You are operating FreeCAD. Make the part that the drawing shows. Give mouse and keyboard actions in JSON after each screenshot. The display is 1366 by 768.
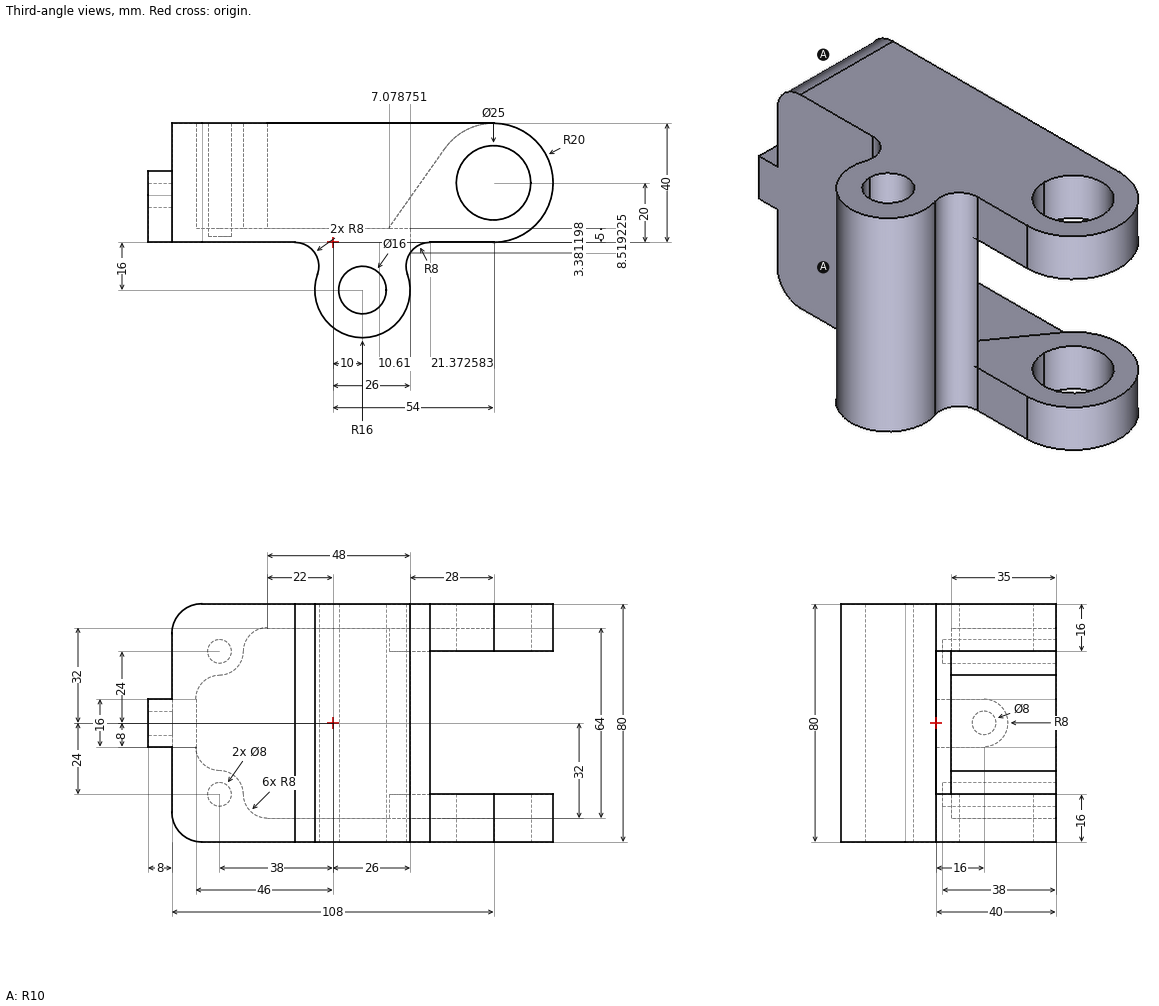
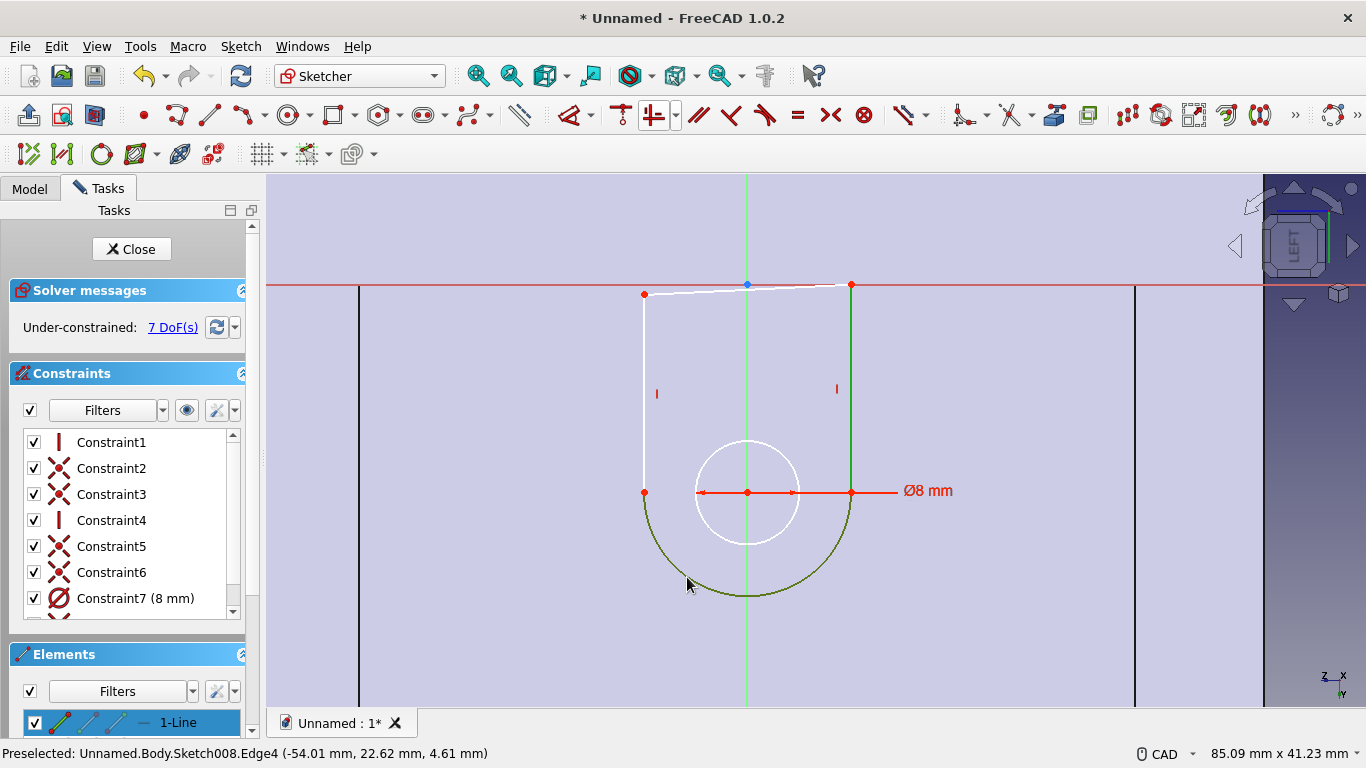
{"action": "key", "text": "t"}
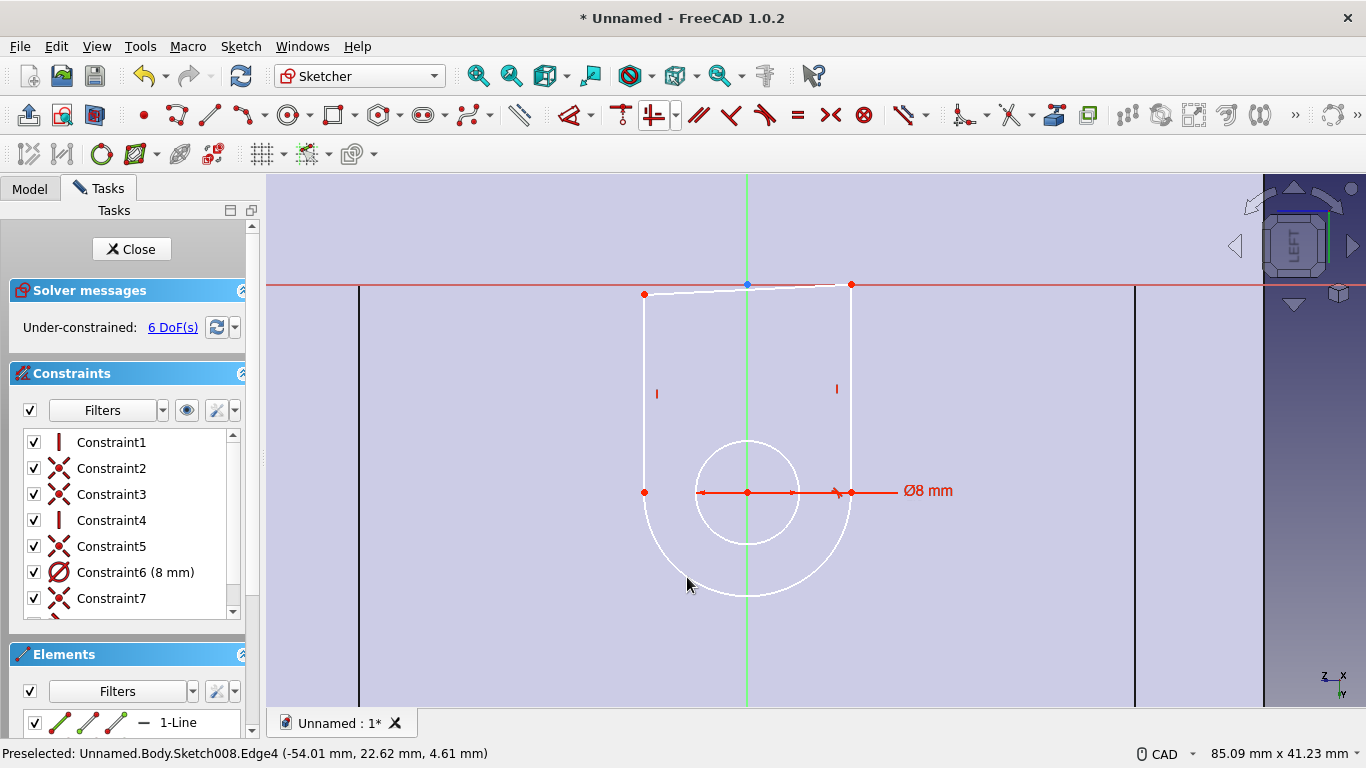
{"action": "left_click", "coordinate": [644, 354]}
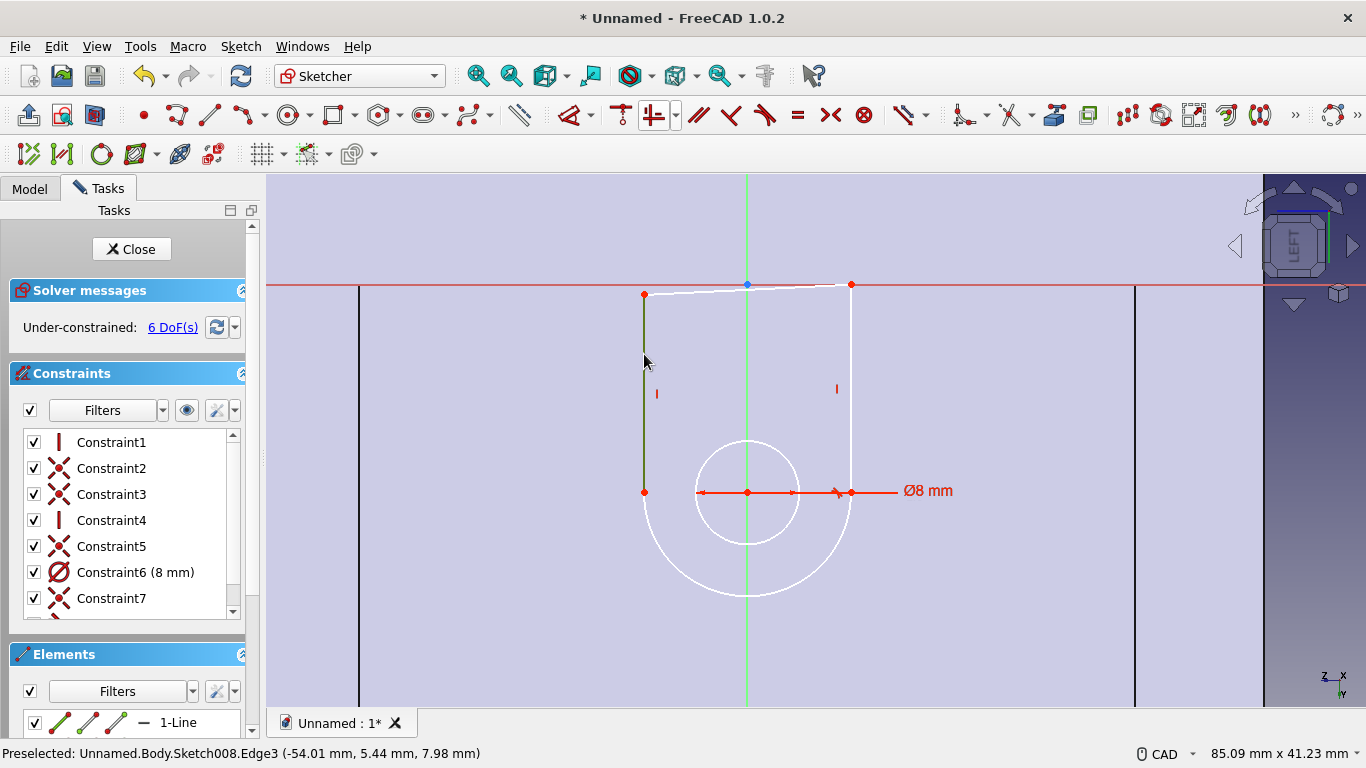
{"action": "left_click", "coordinate": [687, 577]}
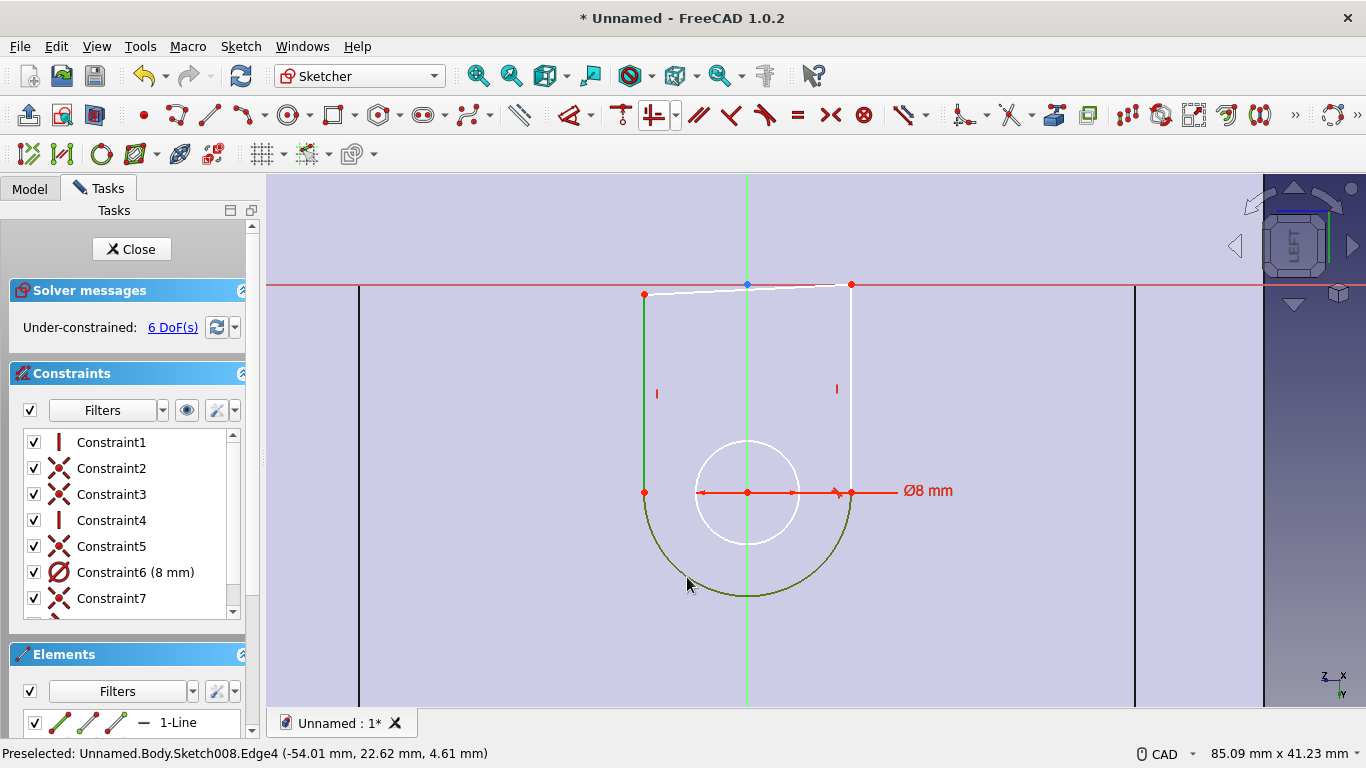
{"action": "key", "text": "t"}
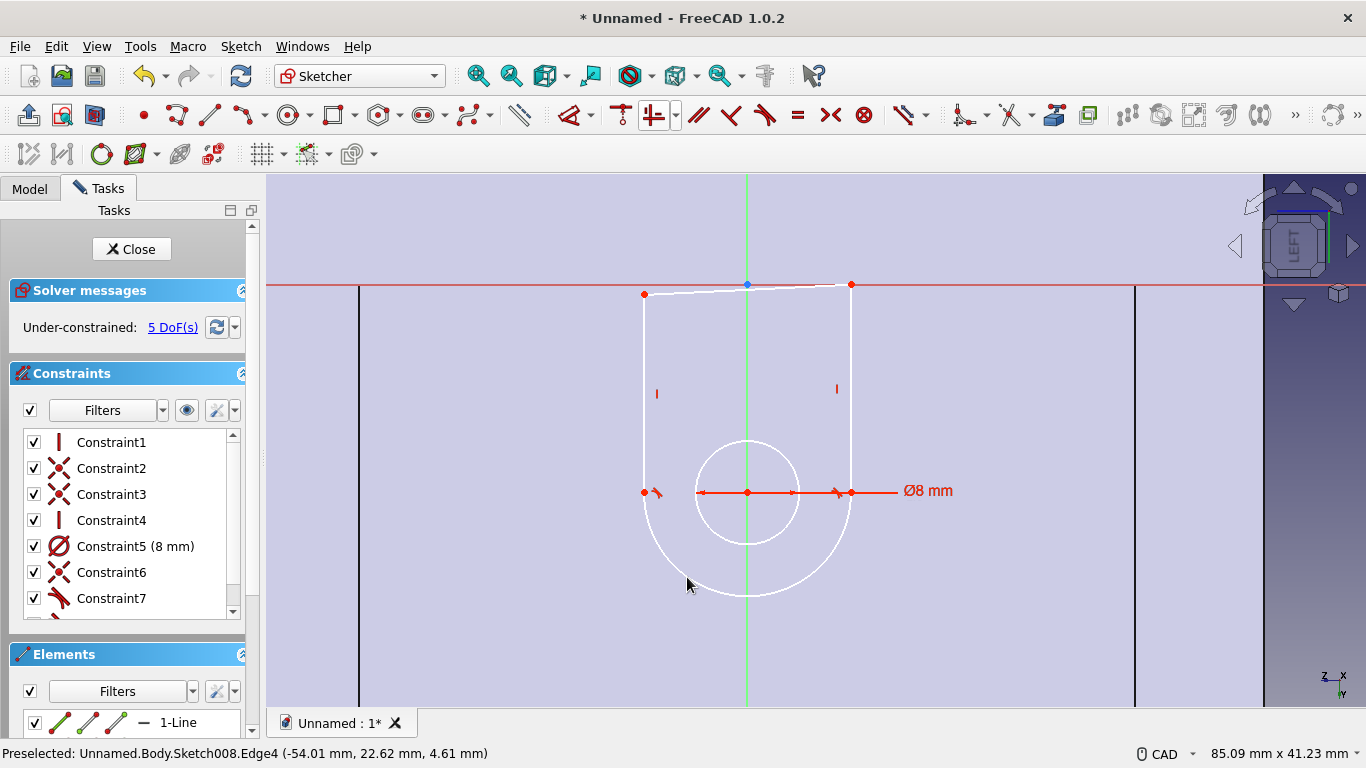
{"action": "left_click", "coordinate": [789, 288]}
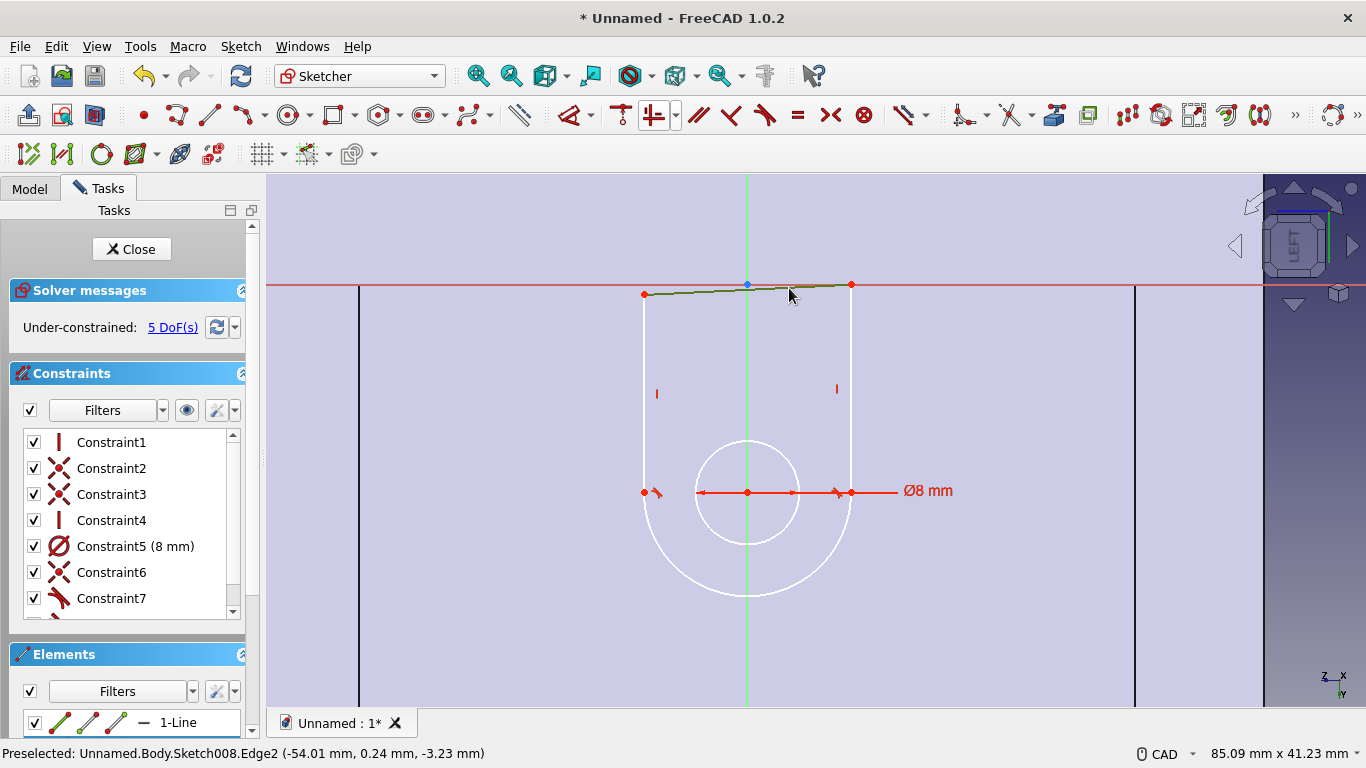
{"action": "key", "text": "h"}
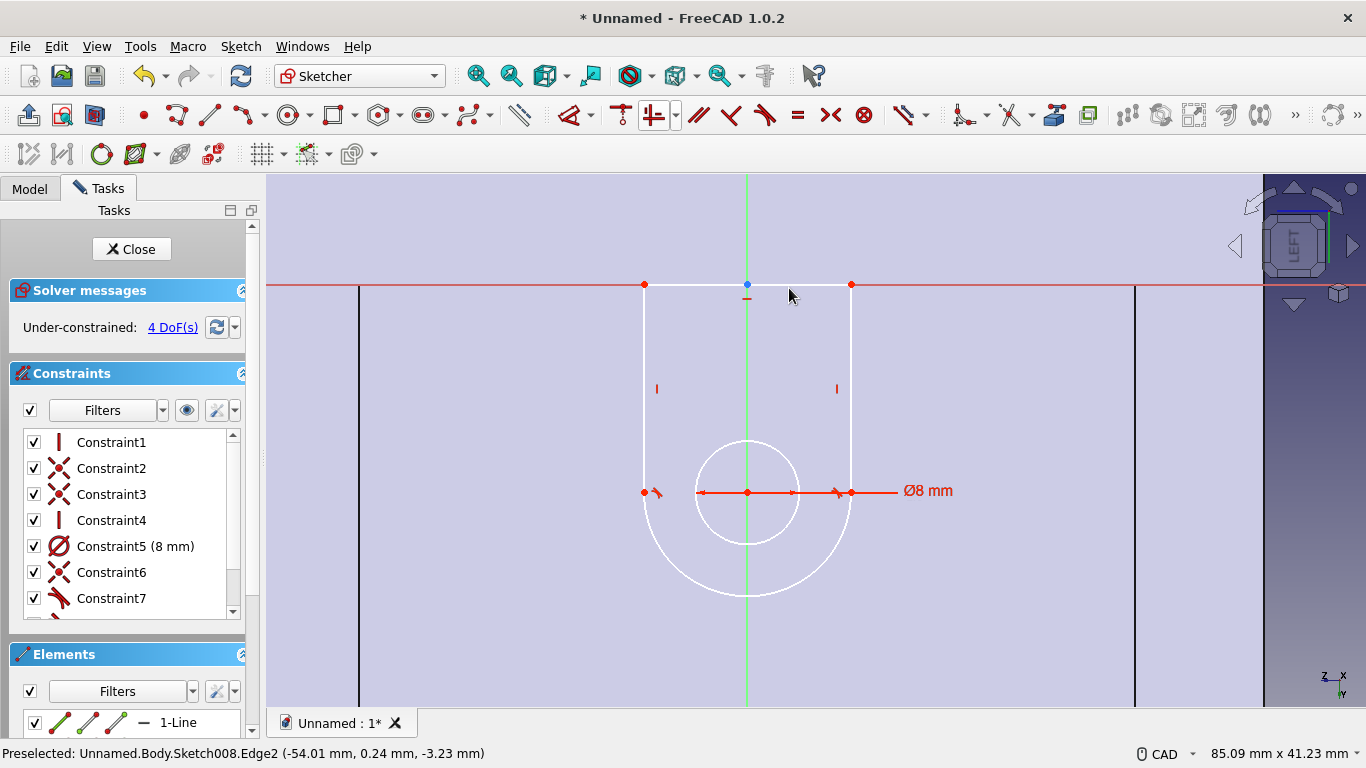
{"action": "left_click", "coordinate": [748, 493]}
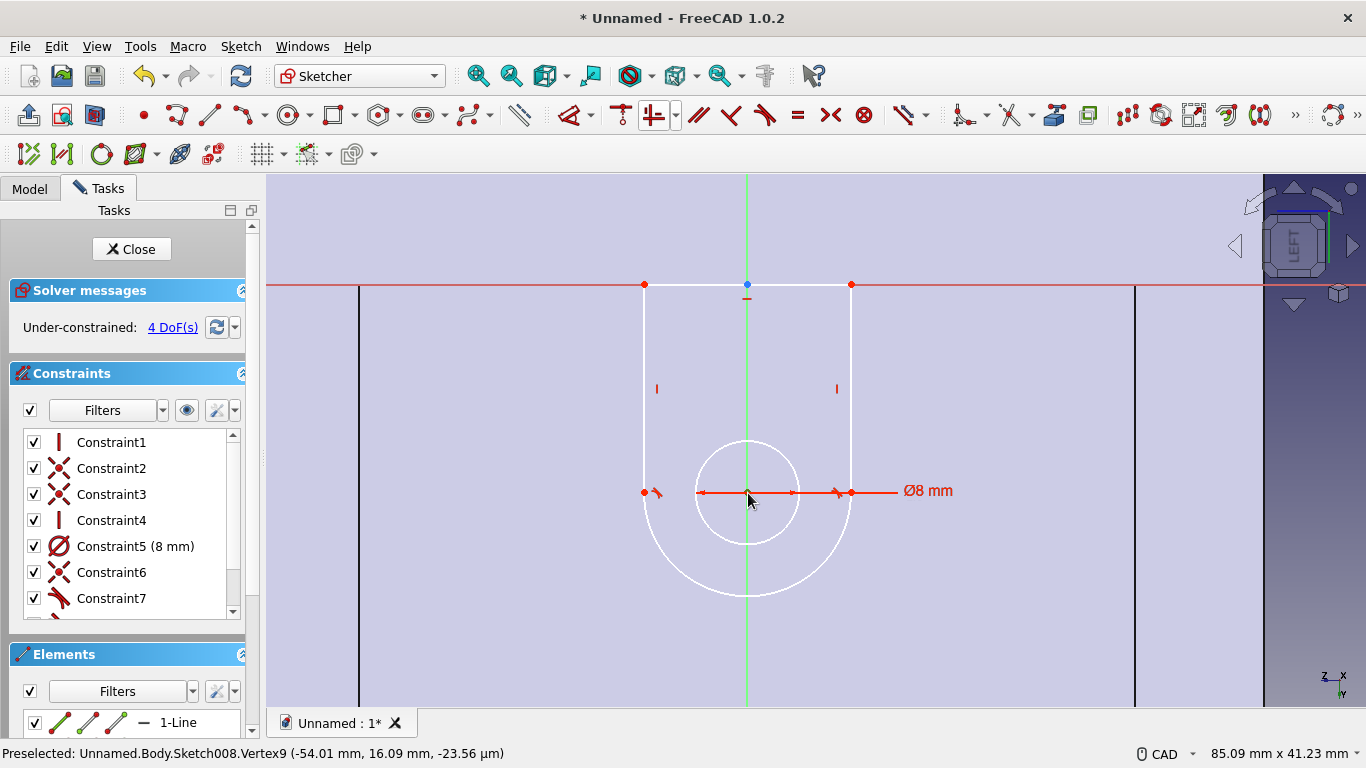
{"action": "left_click", "coordinate": [747, 645]}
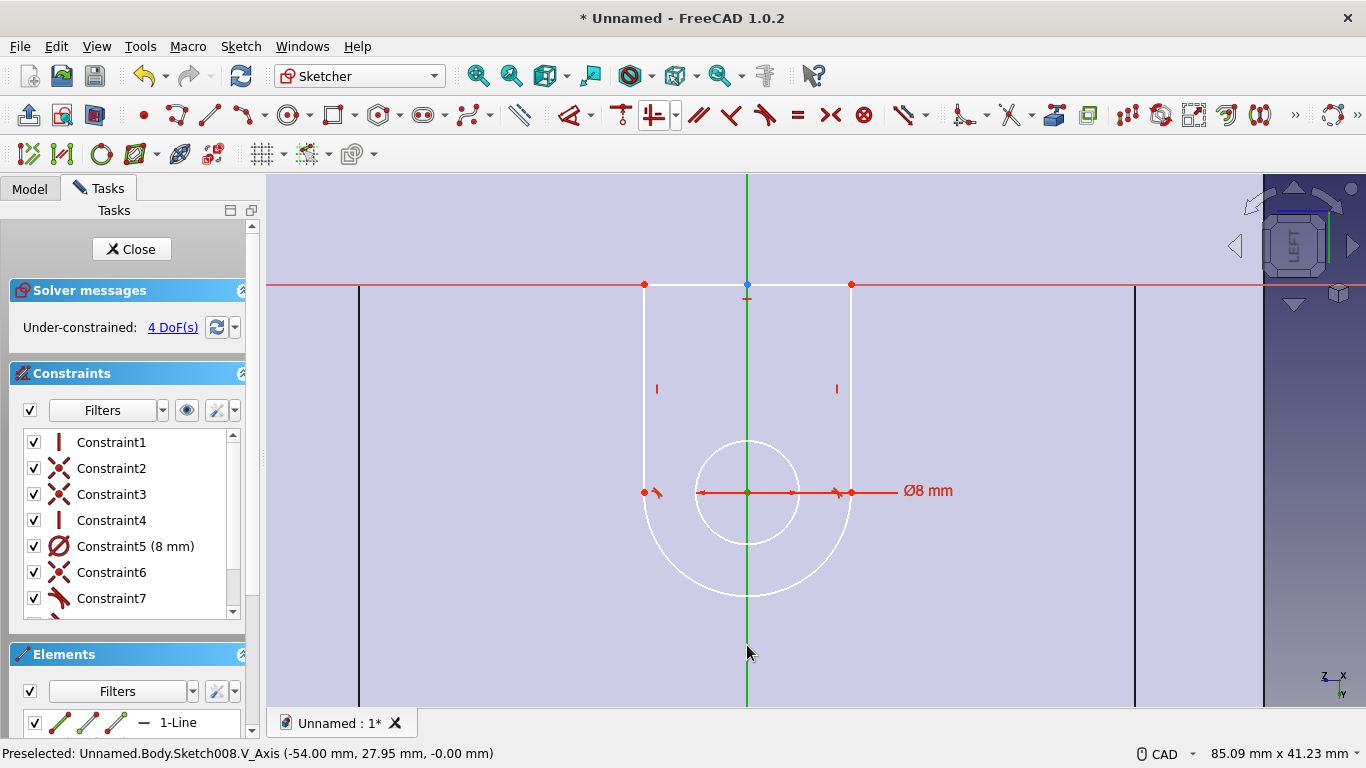
{"action": "left_click", "coordinate": [621, 116]}